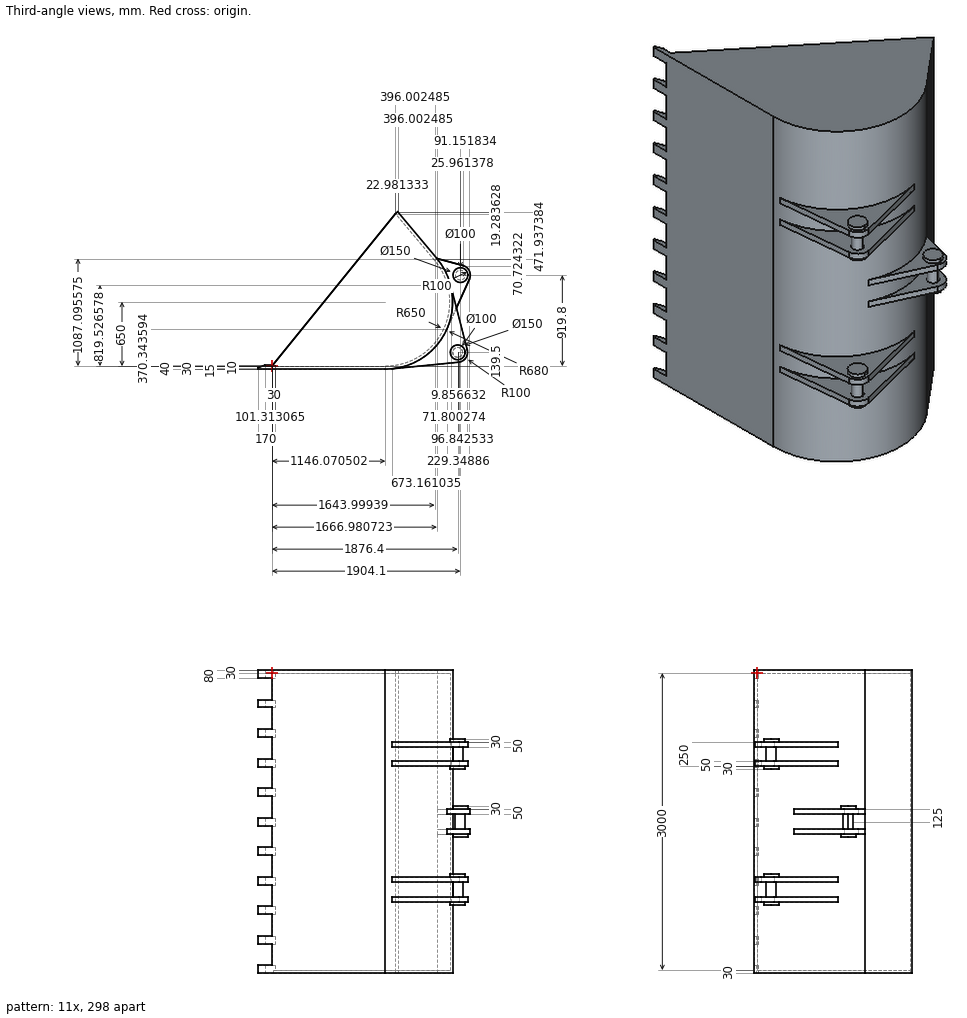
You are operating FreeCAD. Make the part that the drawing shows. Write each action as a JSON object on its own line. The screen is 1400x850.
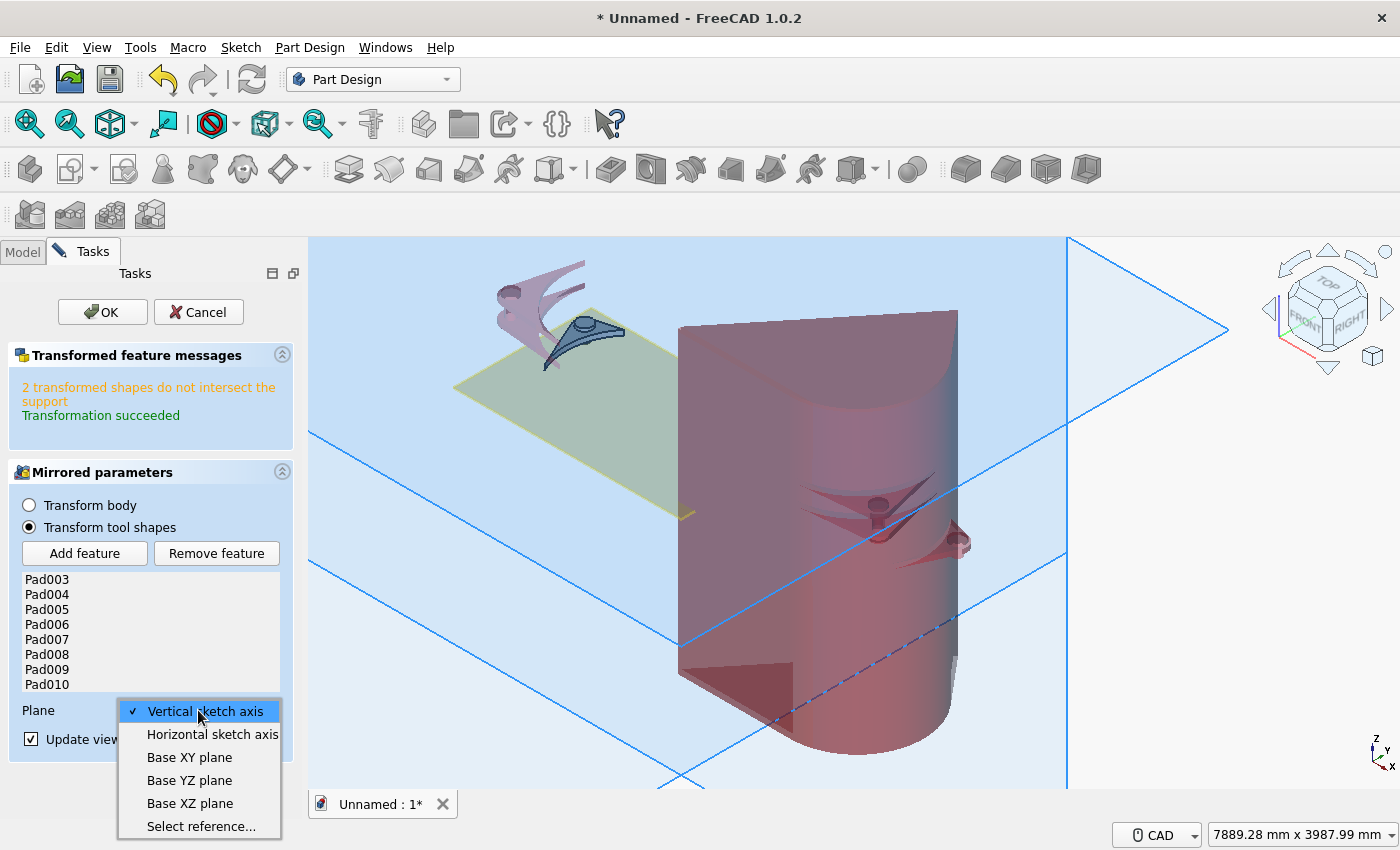
{"action": "left_click", "coordinate": [198, 826]}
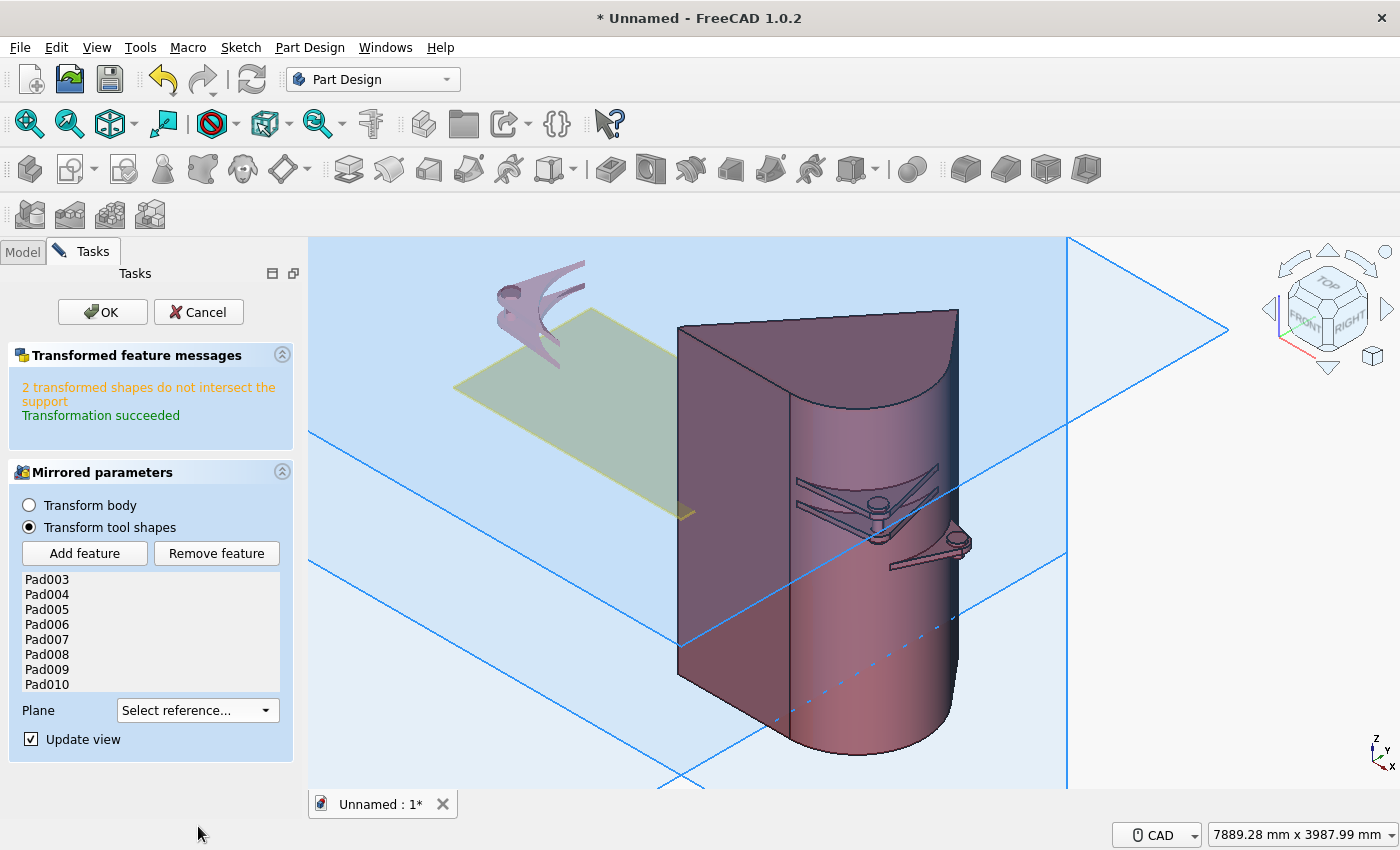
{"action": "left_click", "coordinate": [23, 251]}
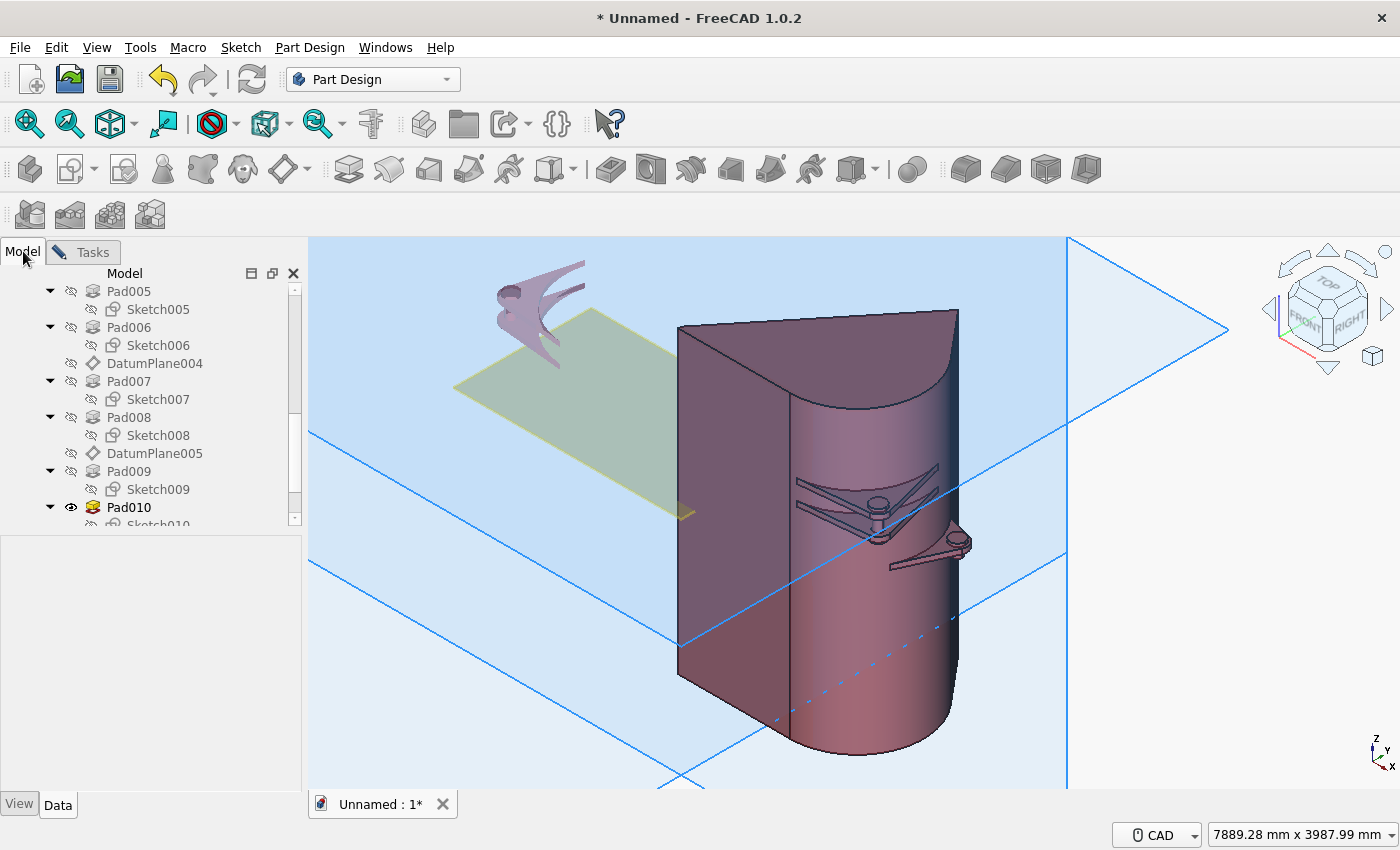
{"action": "scroll", "coordinate": [140, 413], "scroll_direction": "down", "scroll_amount": 3}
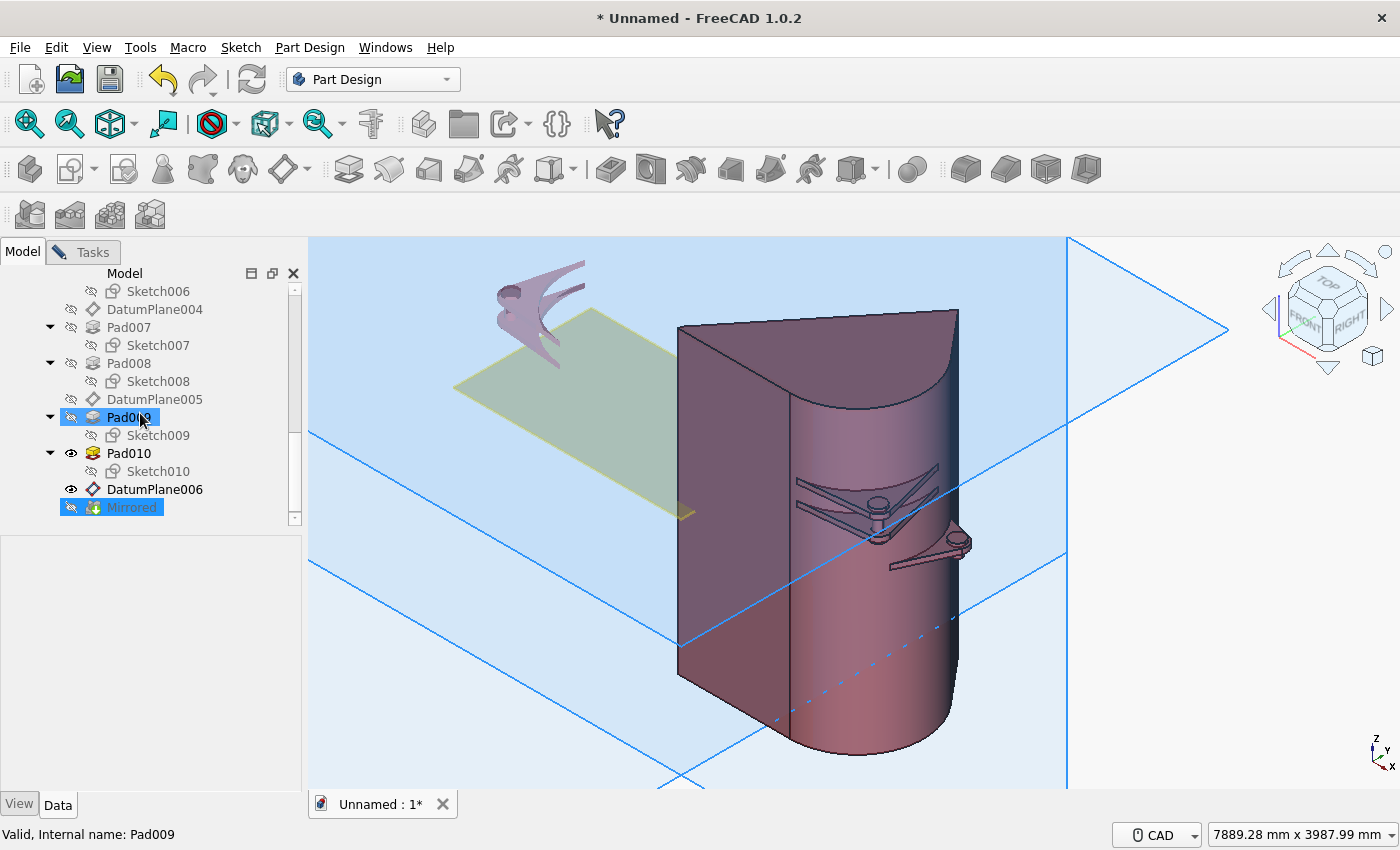
{"action": "left_click", "coordinate": [116, 489]}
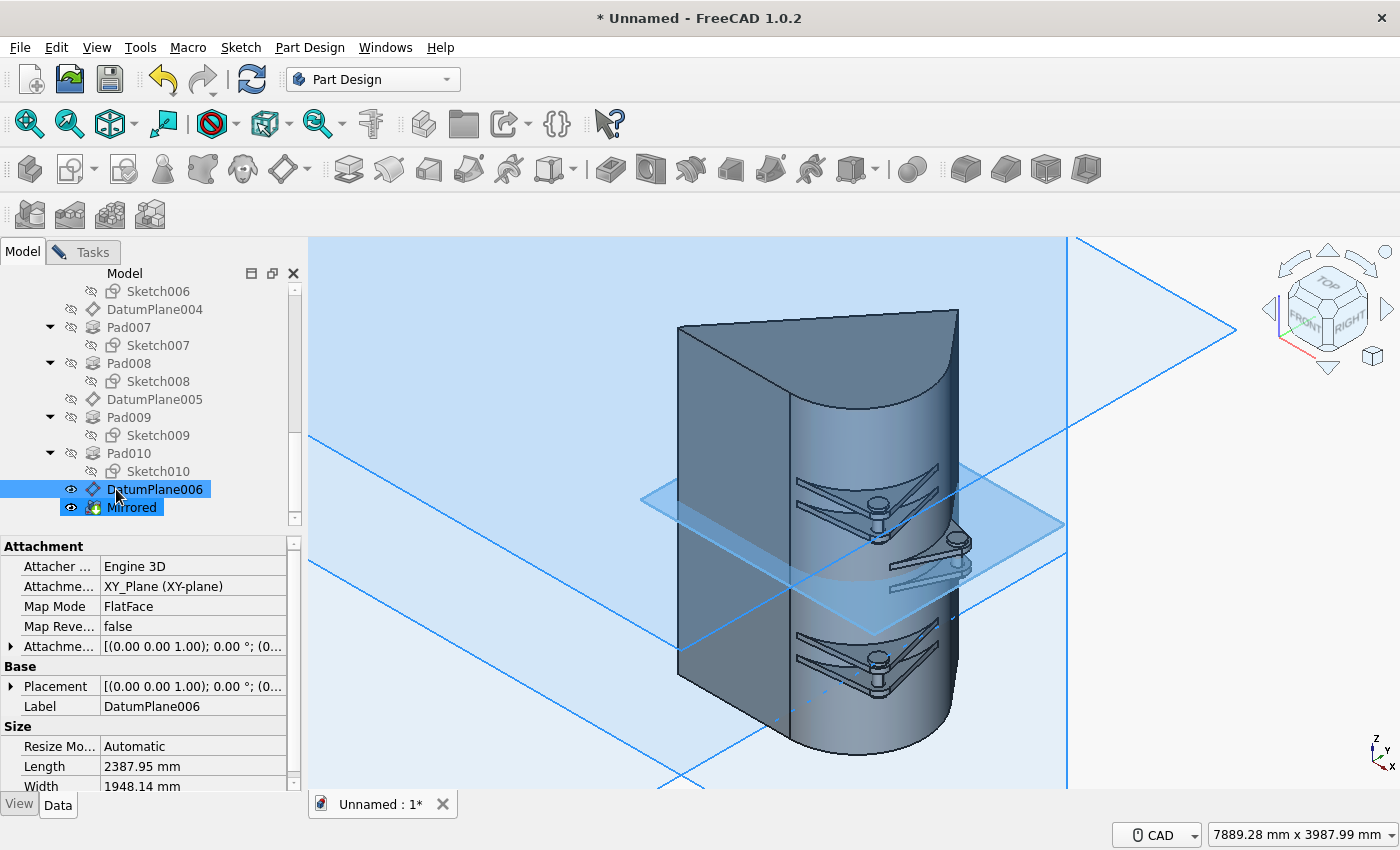
{"action": "left_click", "coordinate": [84, 251]}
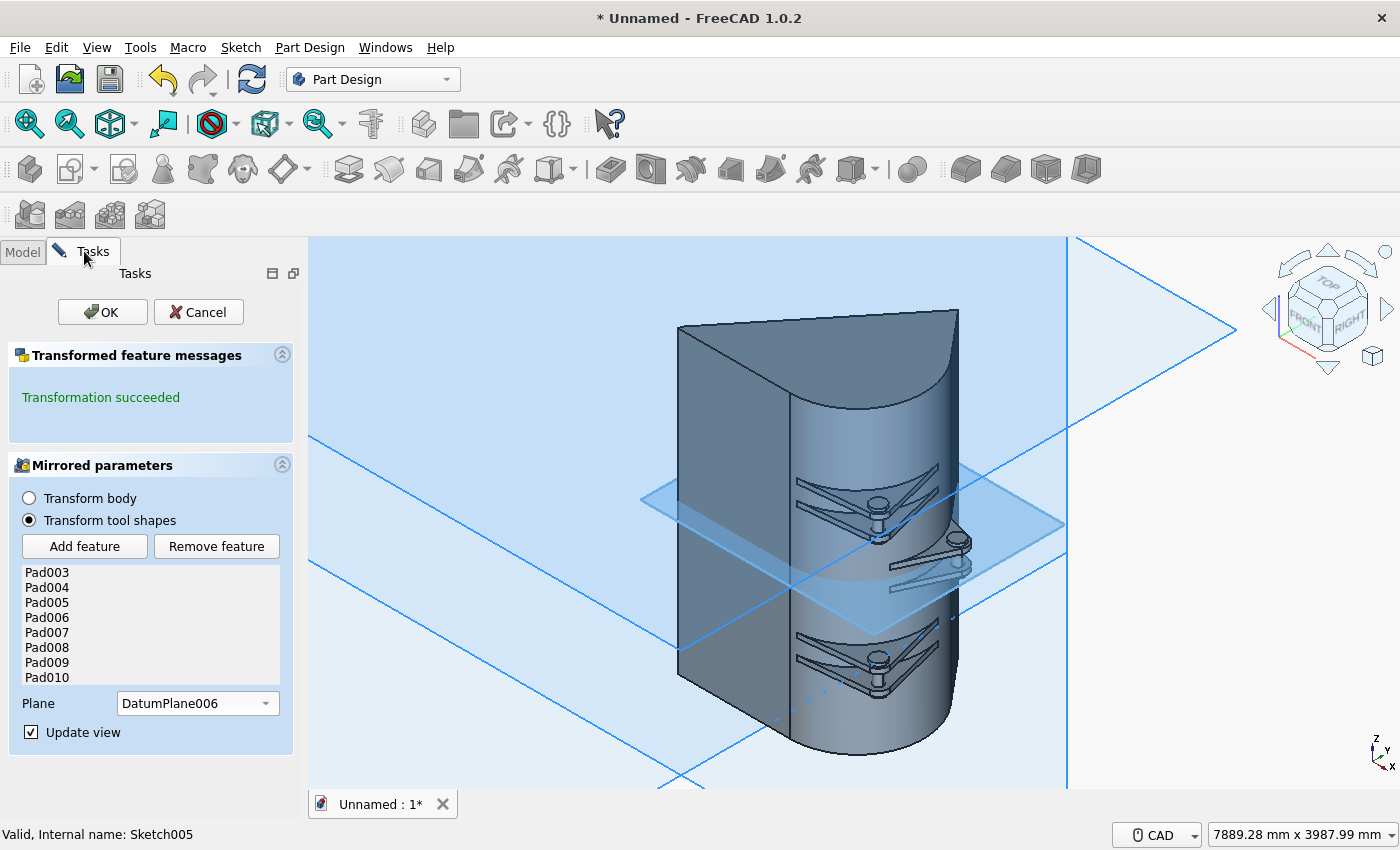
{"action": "left_click", "coordinate": [103, 312]}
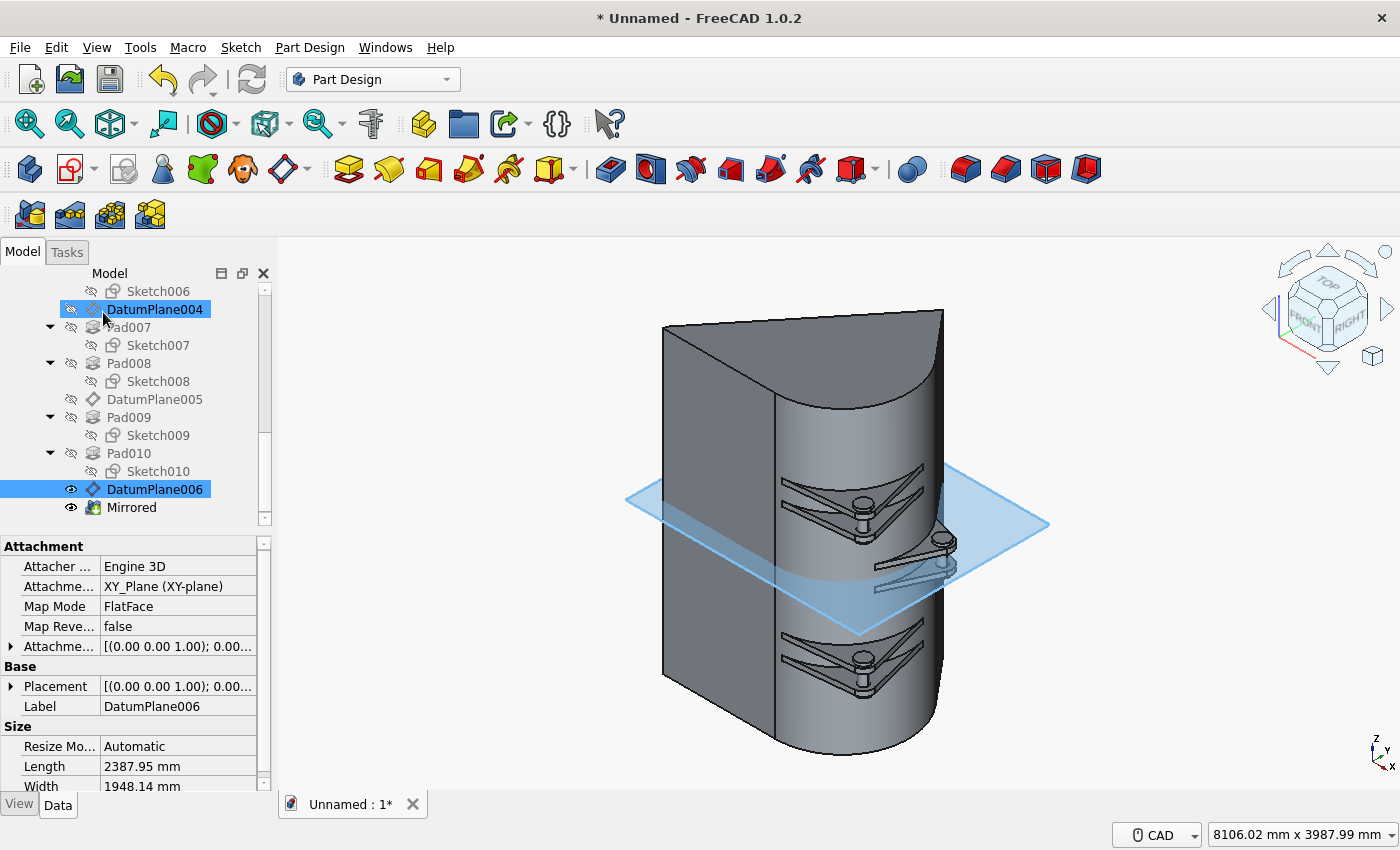
{"action": "left_click", "coordinate": [116, 489]}
{"action": "key", "text": "space"}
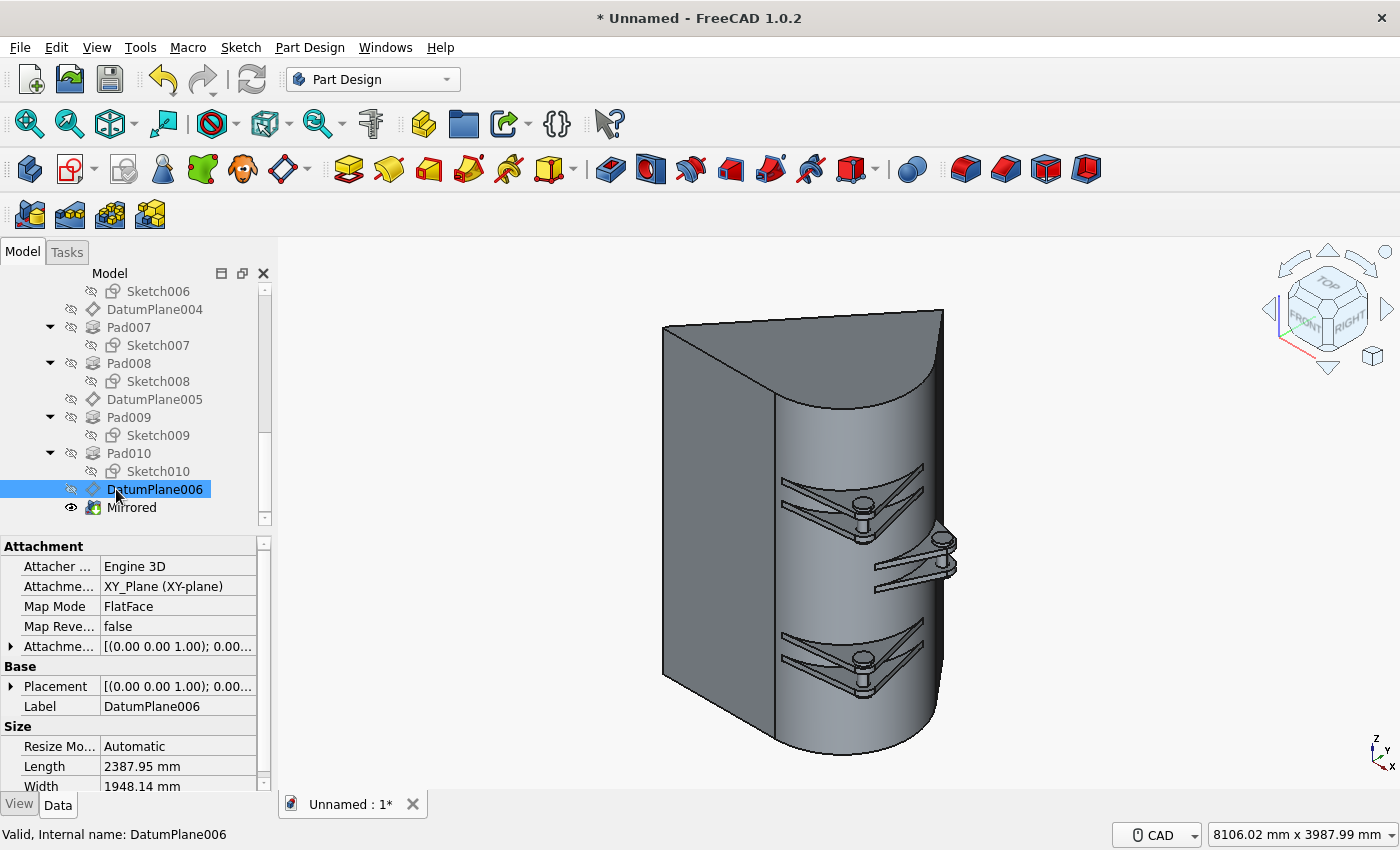
{"action": "left_click", "coordinate": [834, 362]}